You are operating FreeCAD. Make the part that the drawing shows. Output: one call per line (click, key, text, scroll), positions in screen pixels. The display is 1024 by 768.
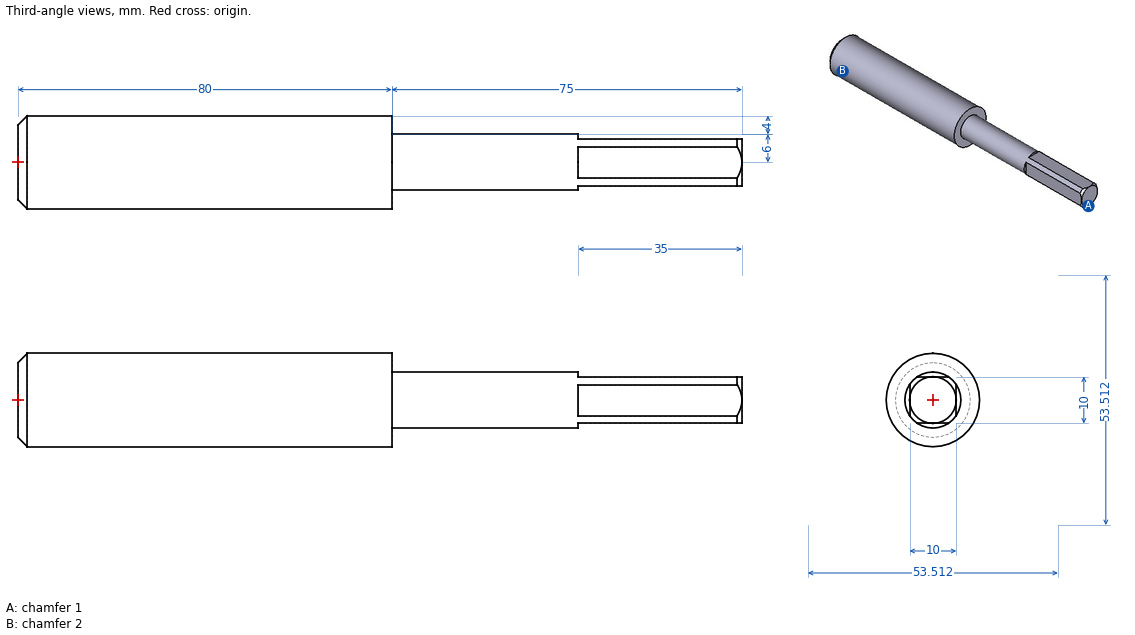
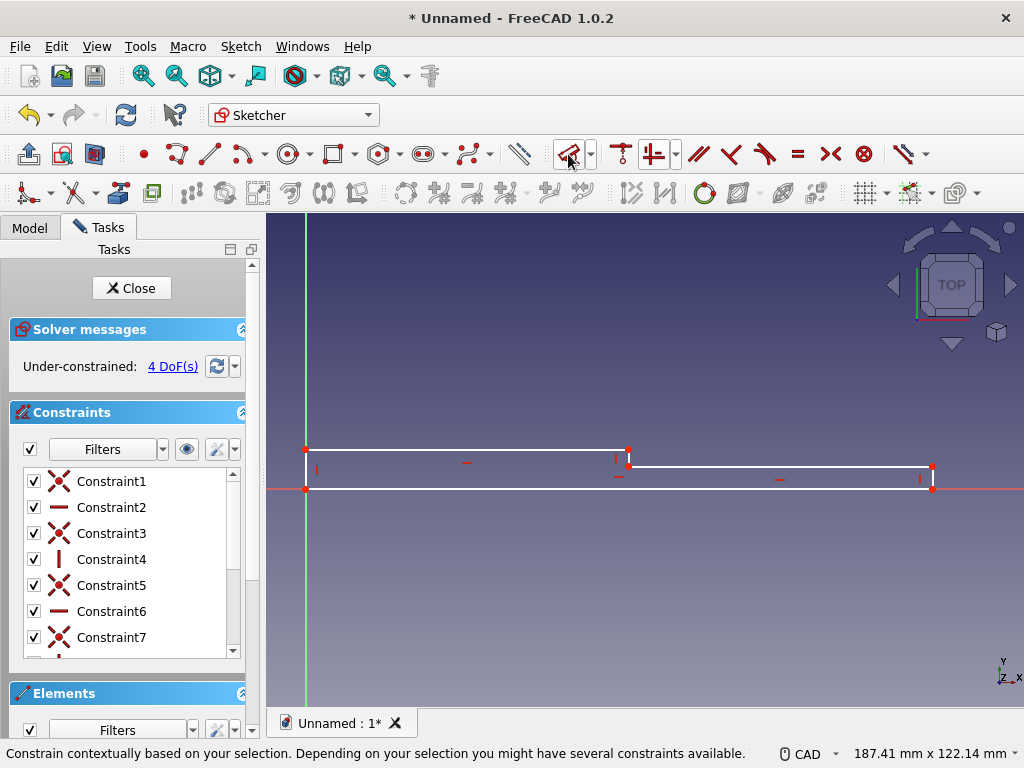
scroll(490, 442, down, 2)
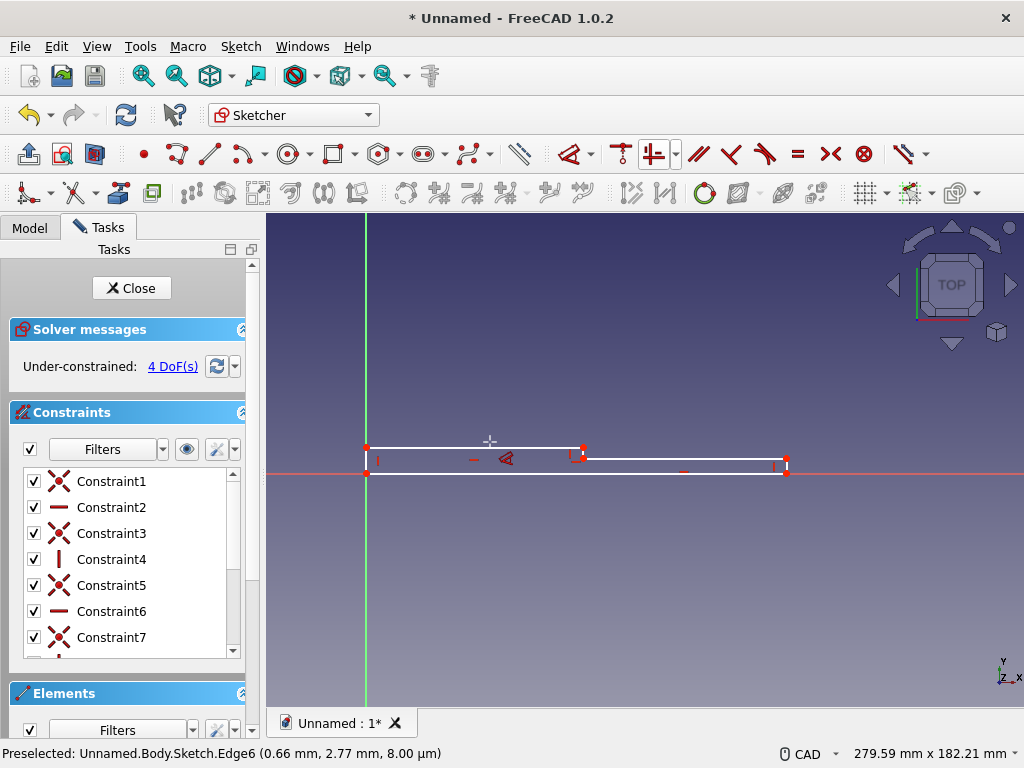
scroll(787, 466, up, 5)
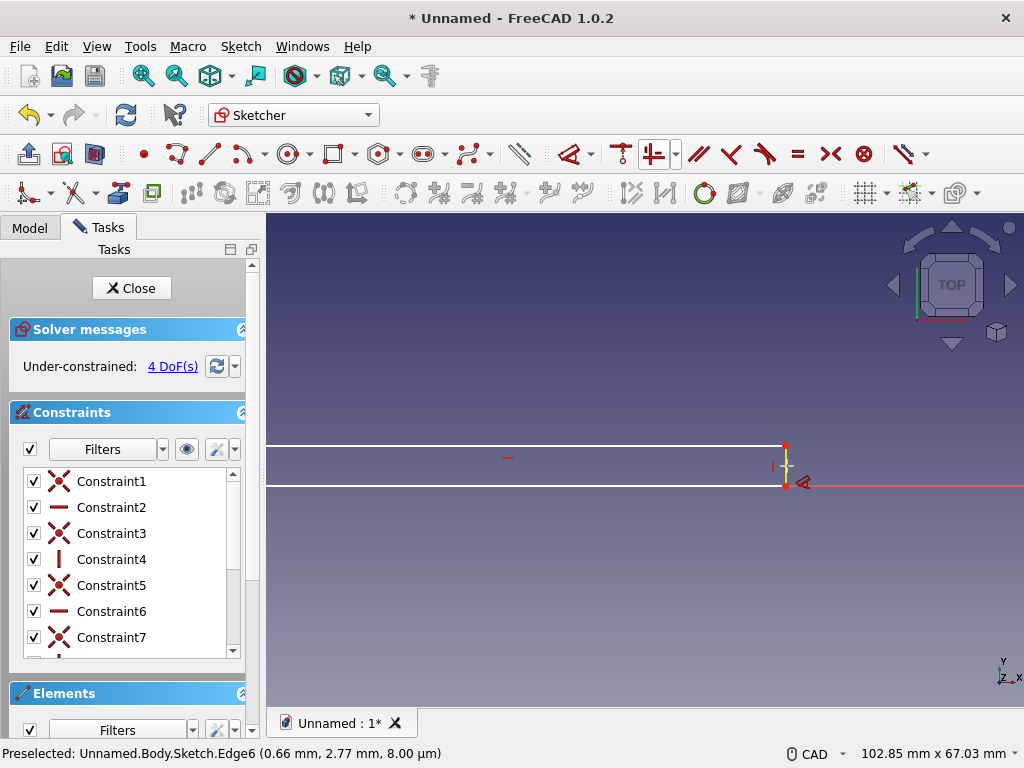
click(786, 466)
click(820, 466)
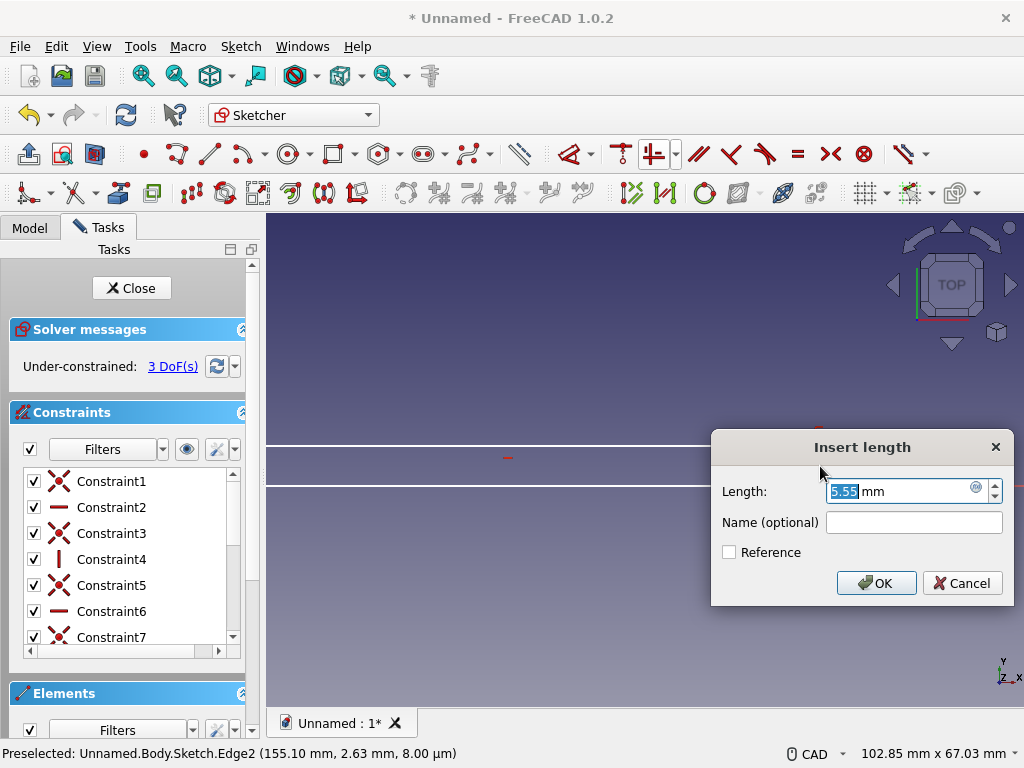
text(6)
key(Return)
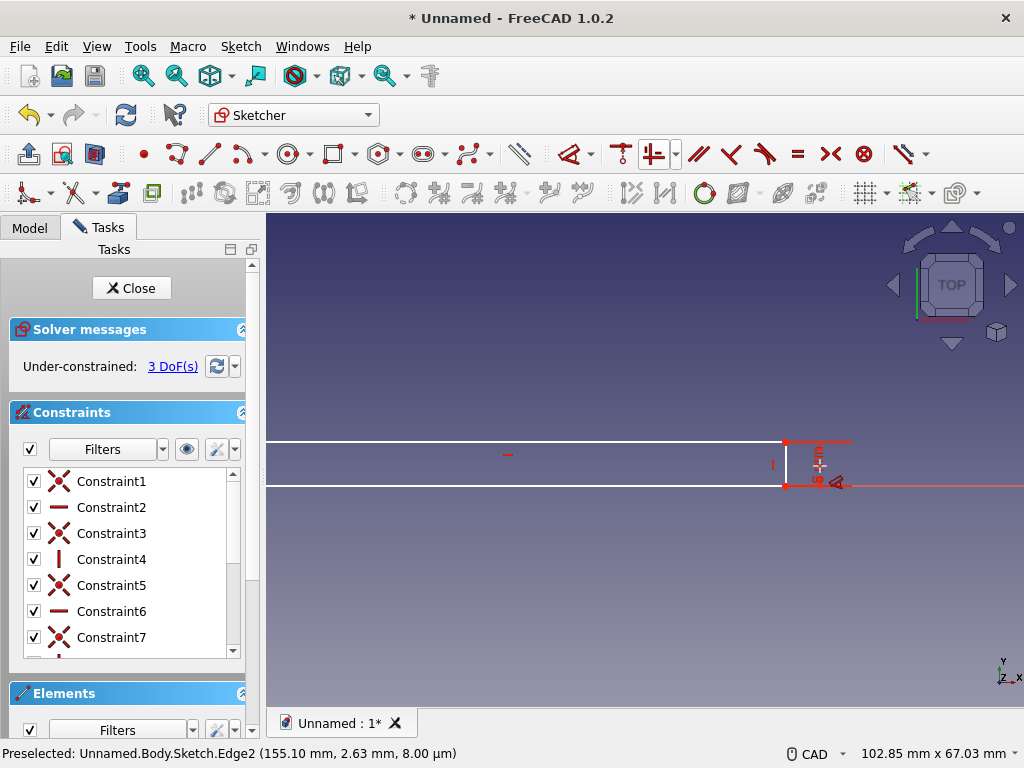
scroll(788, 466, down, 5)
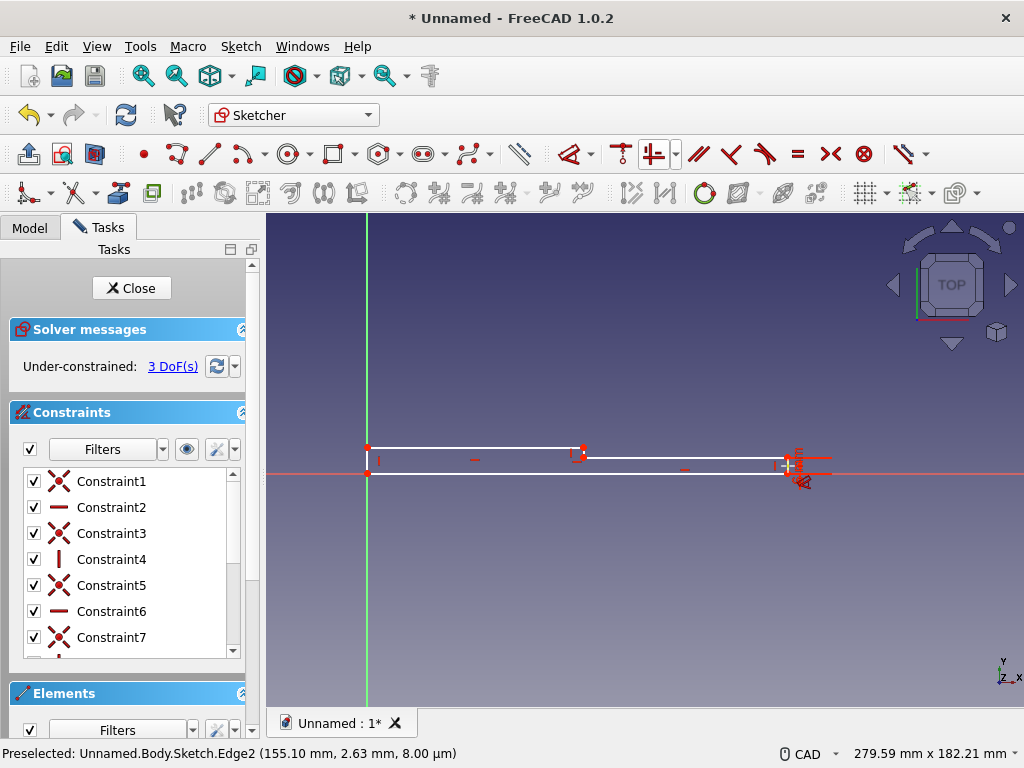
scroll(584, 454, up, 7)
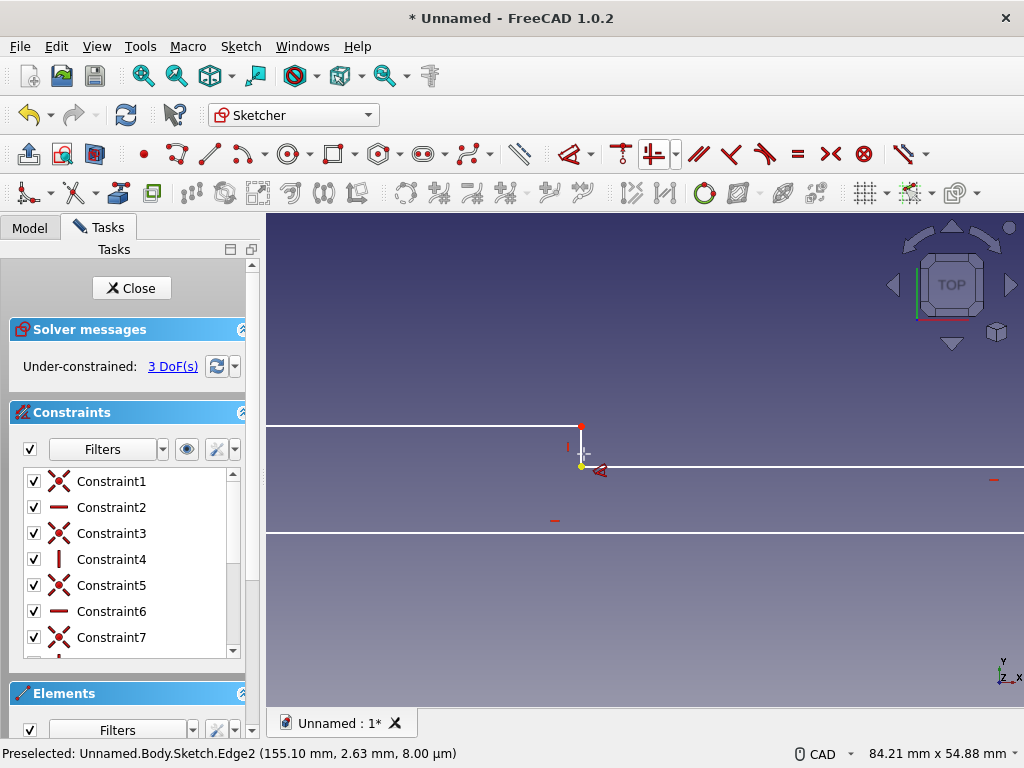
click(581, 451)
click(615, 447)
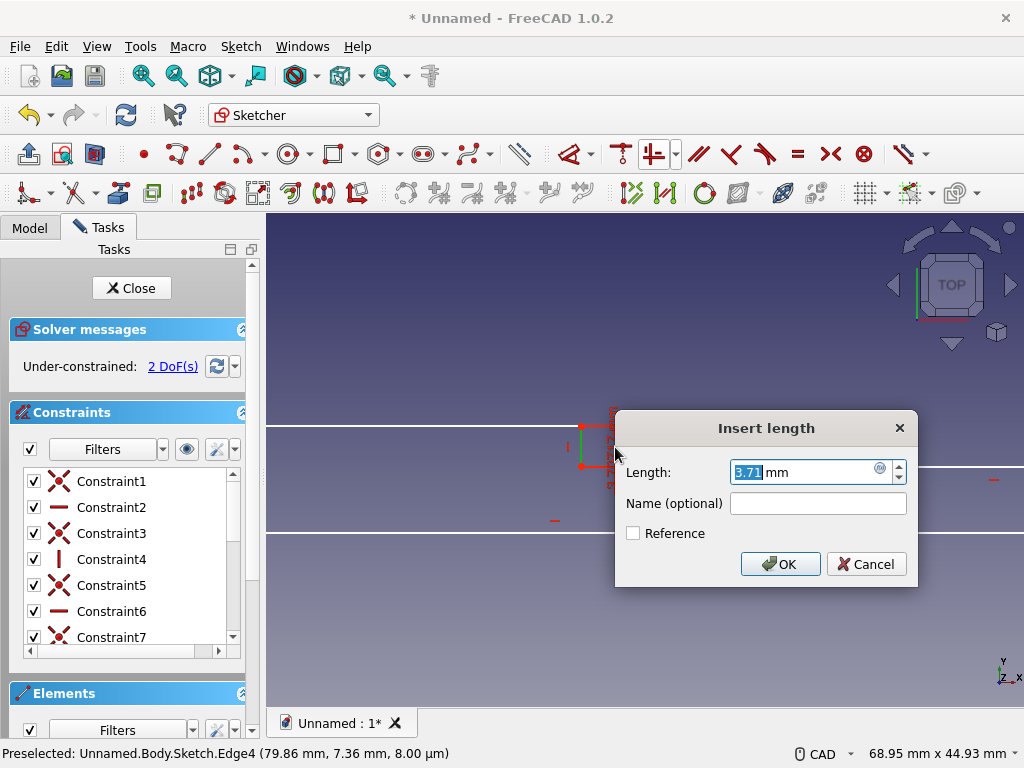
text(4)
key(Return)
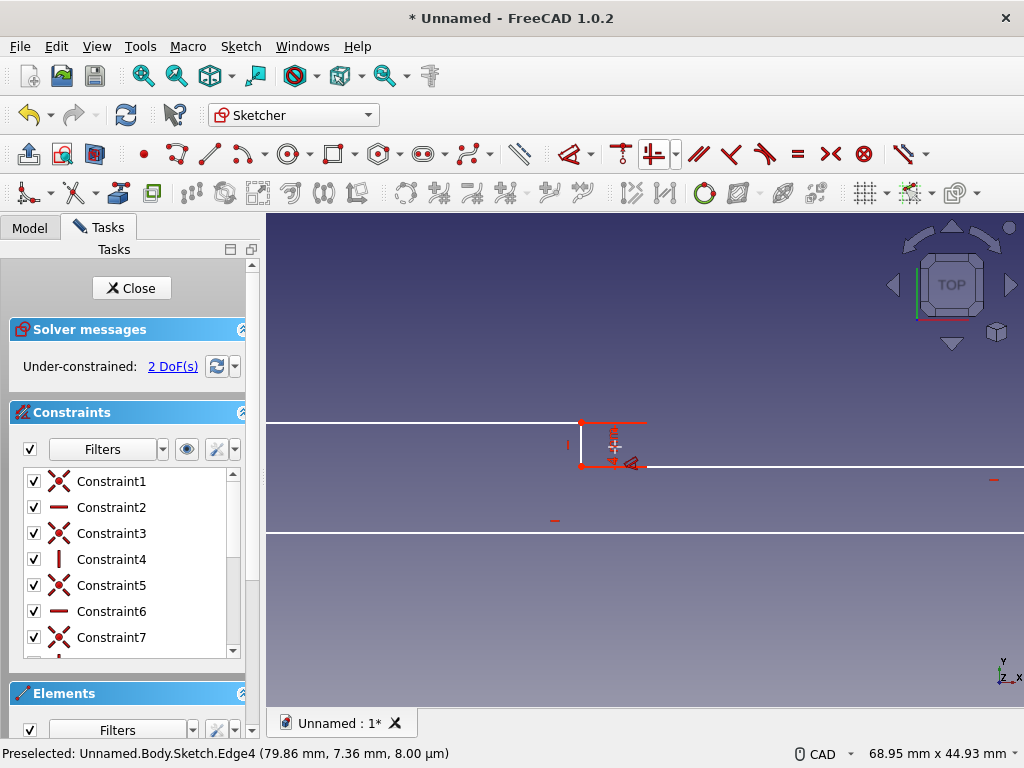
scroll(583, 454, down, 7)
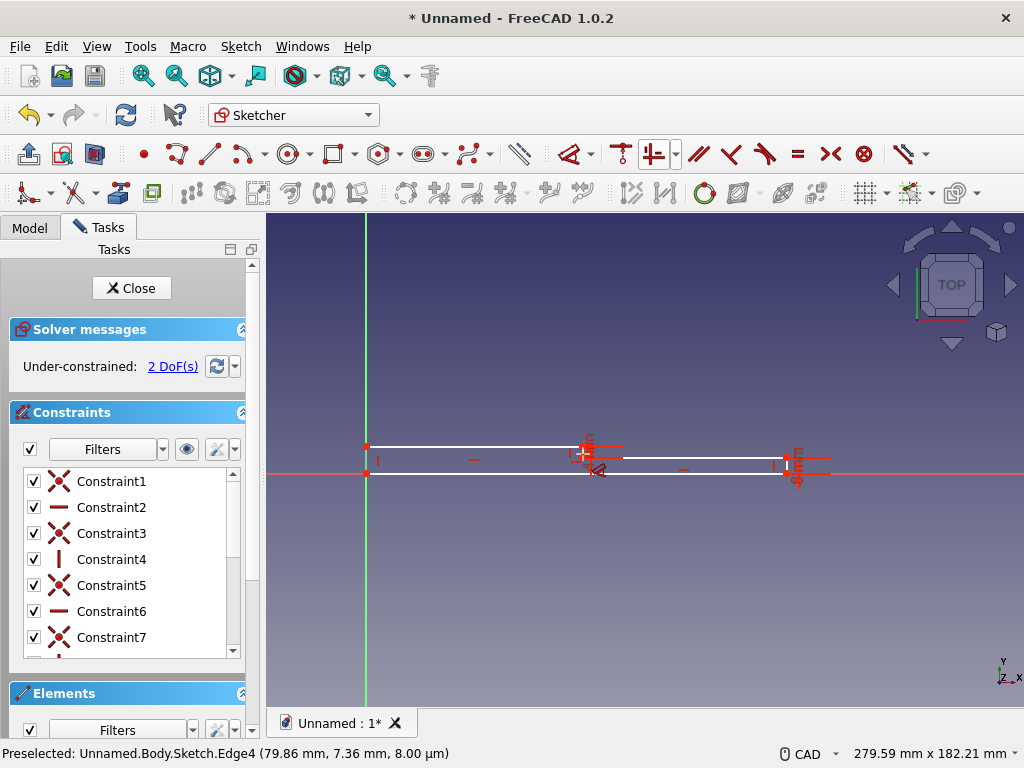
click(644, 458)
click(685, 424)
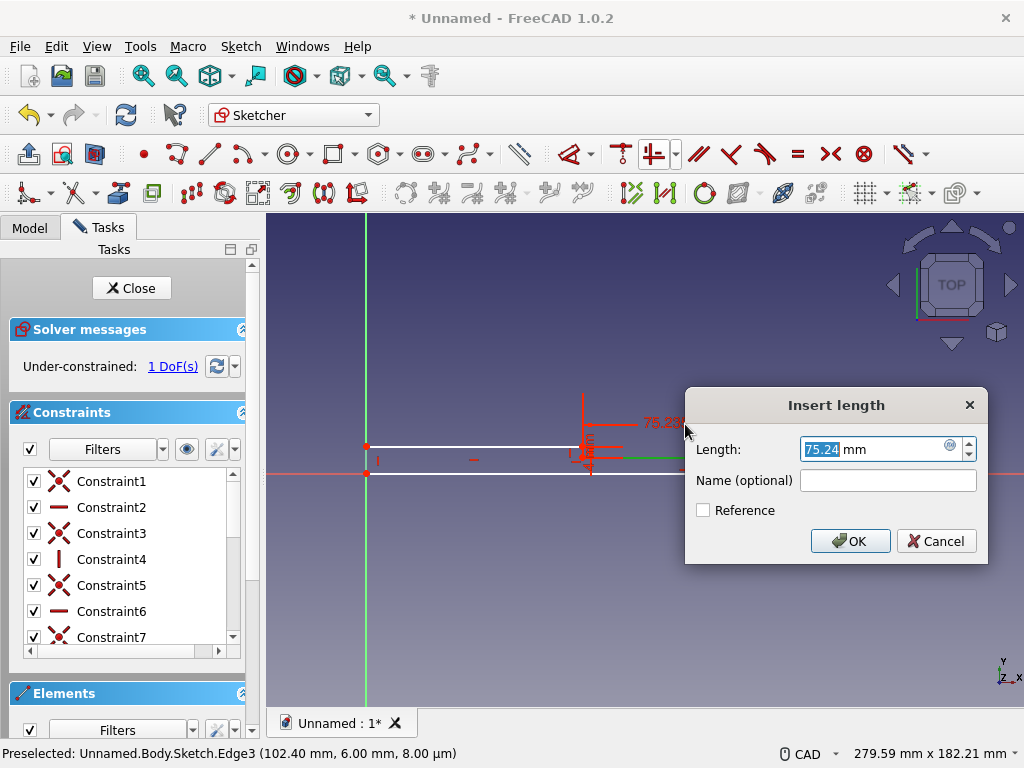
text(75)
key(Return)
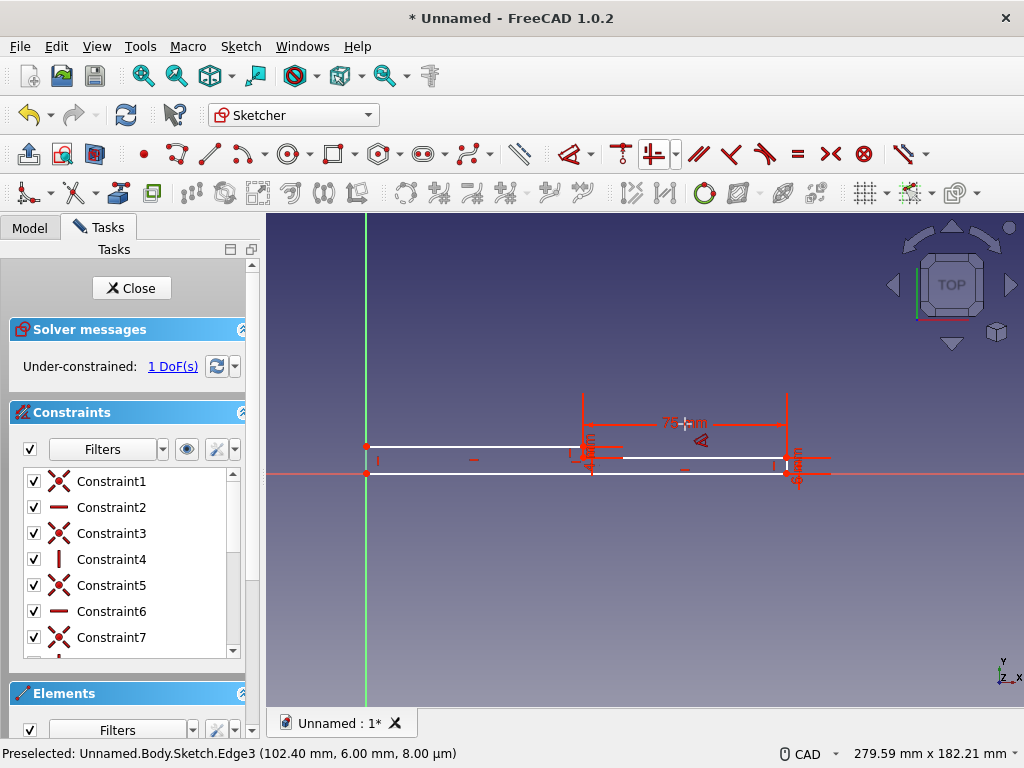
click(518, 447)
click(475, 413)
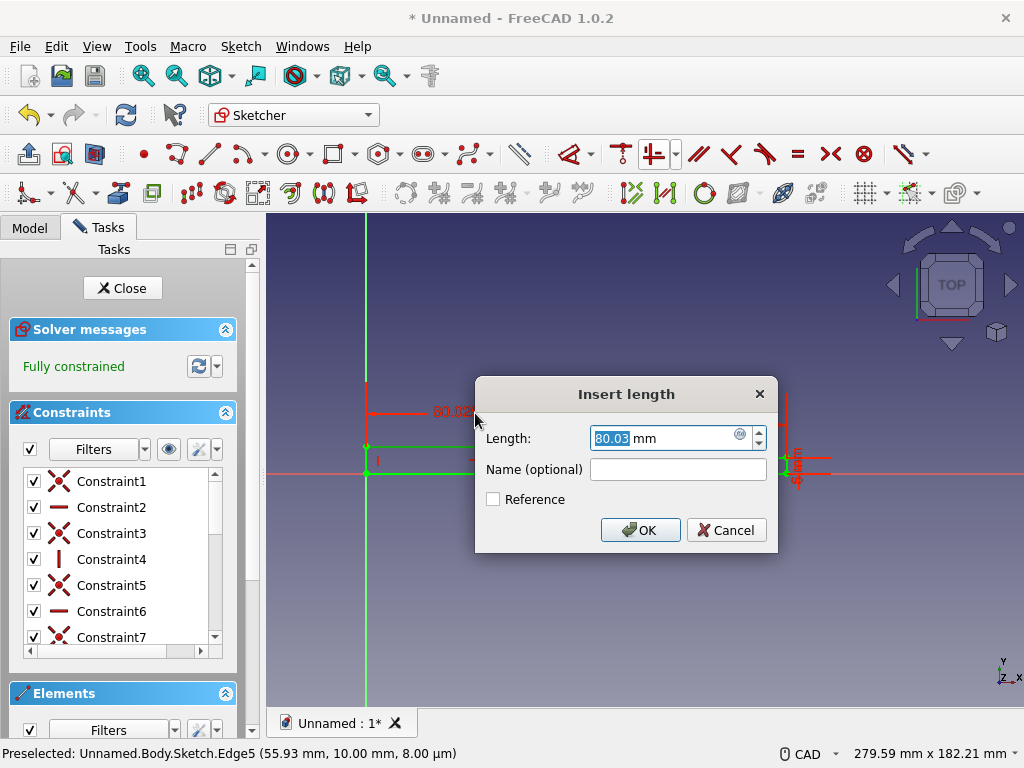
text(80)
key(Return)
key(Escape)